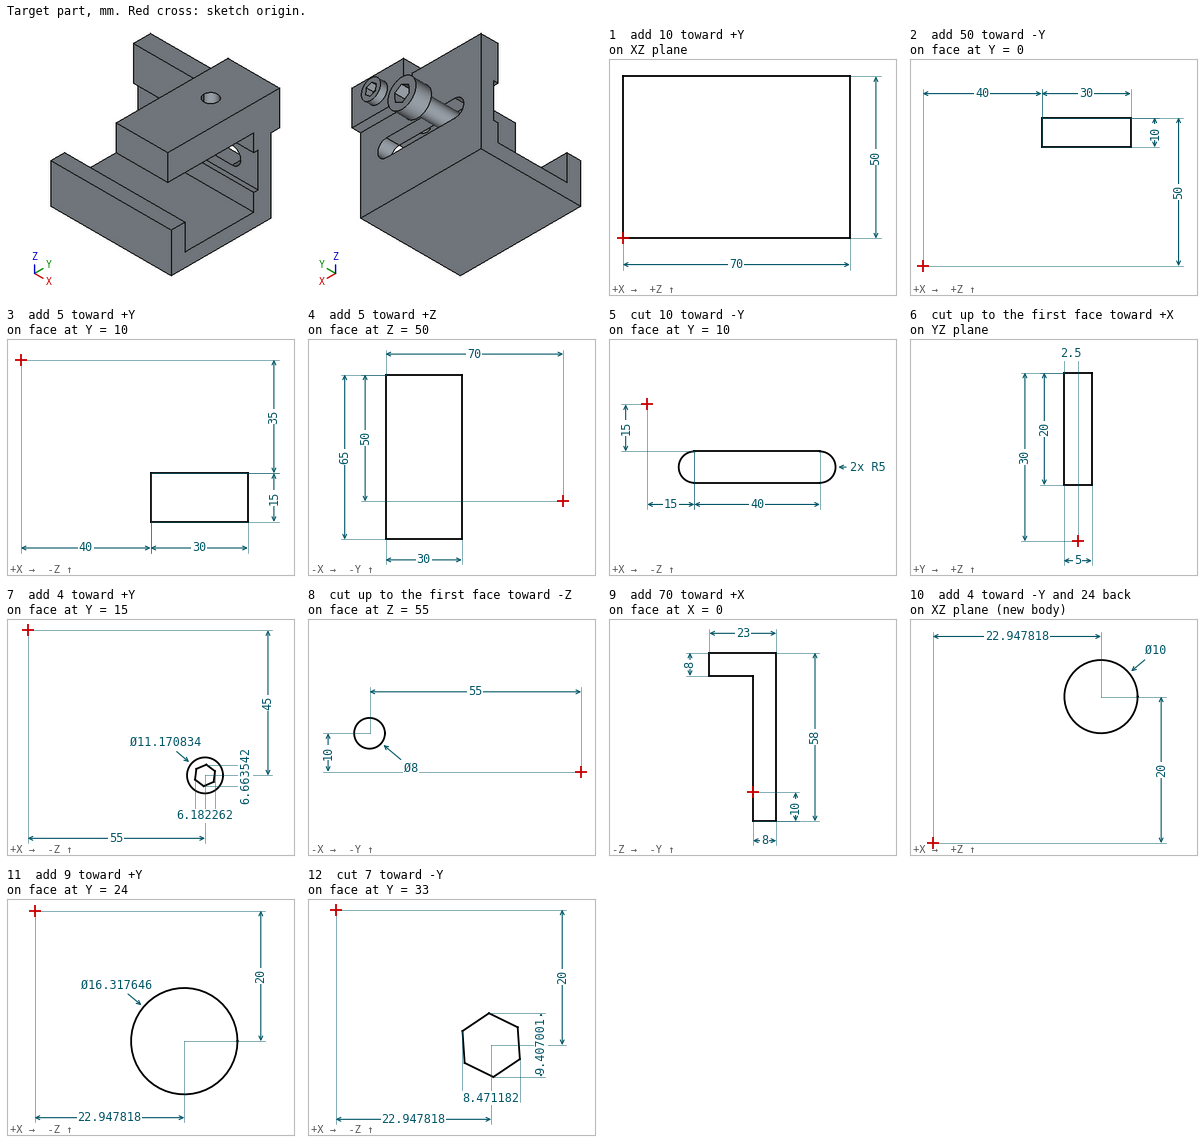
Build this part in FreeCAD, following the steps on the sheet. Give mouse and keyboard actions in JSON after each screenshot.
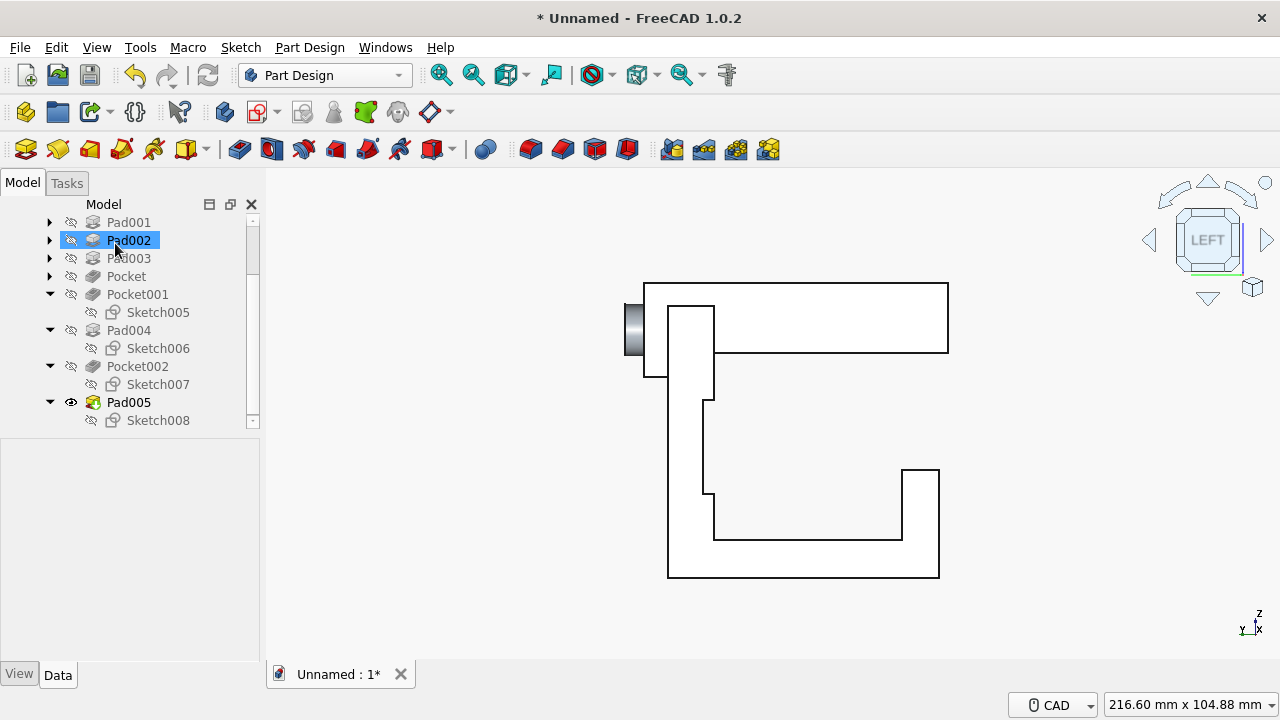
{"action": "left_click", "coordinate": [226, 112]}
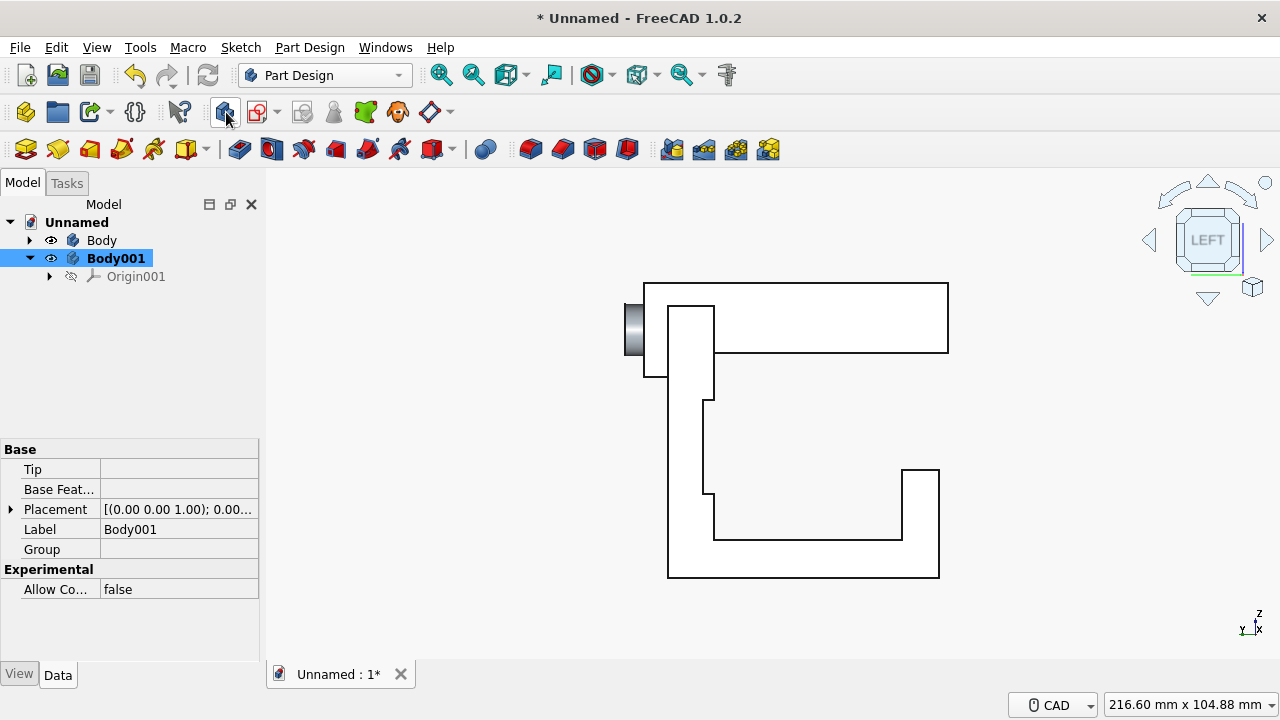
{"action": "left_click", "coordinate": [306, 619]}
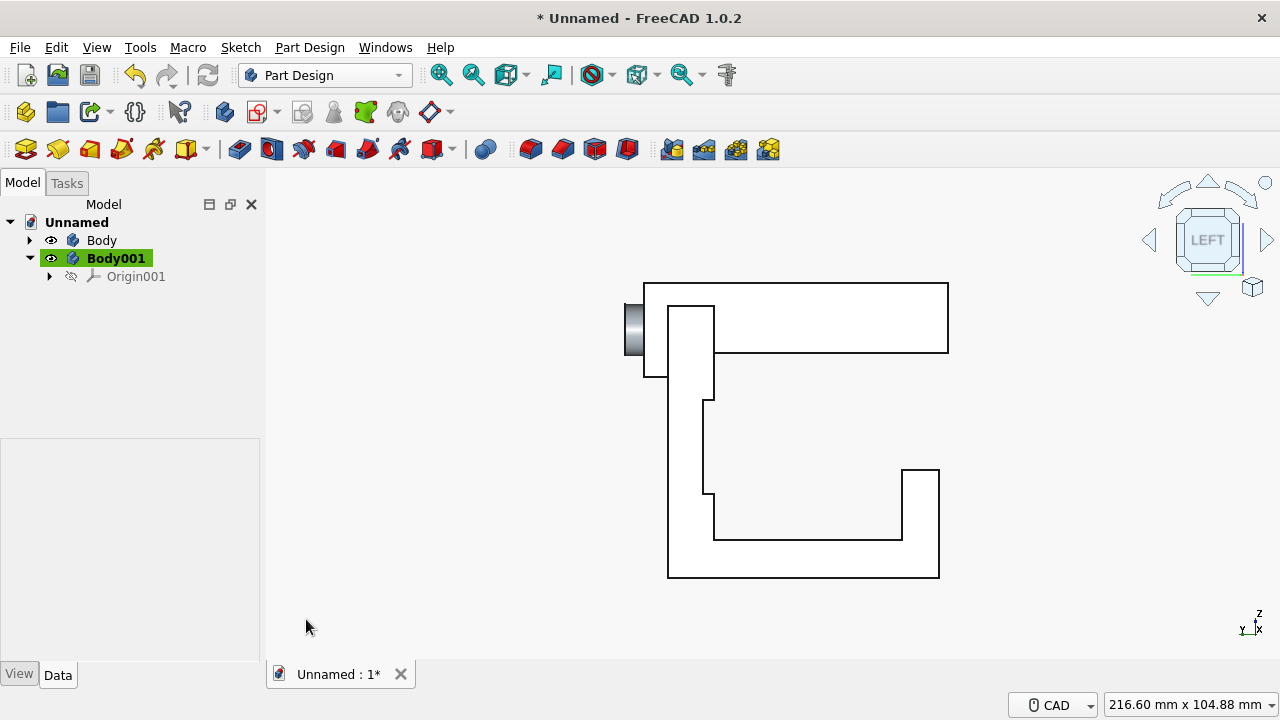
{"action": "left_click", "coordinate": [258, 112]}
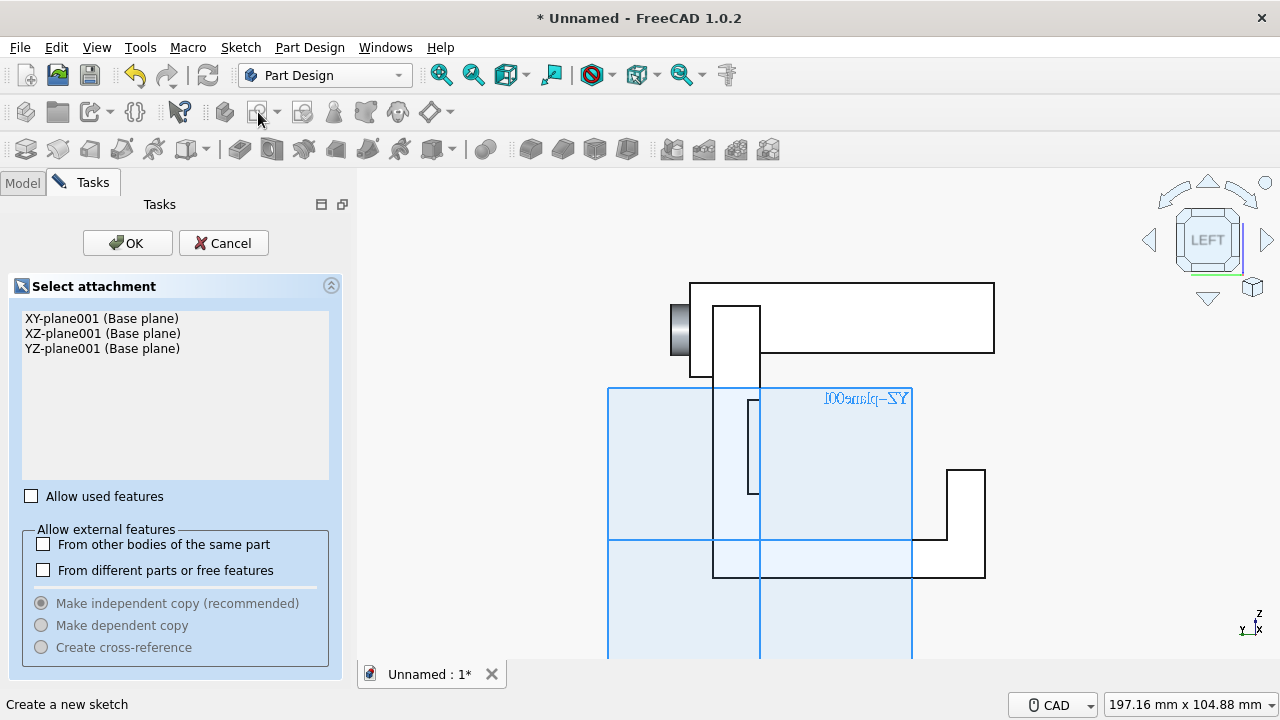
{"action": "left_click", "coordinate": [82, 334]}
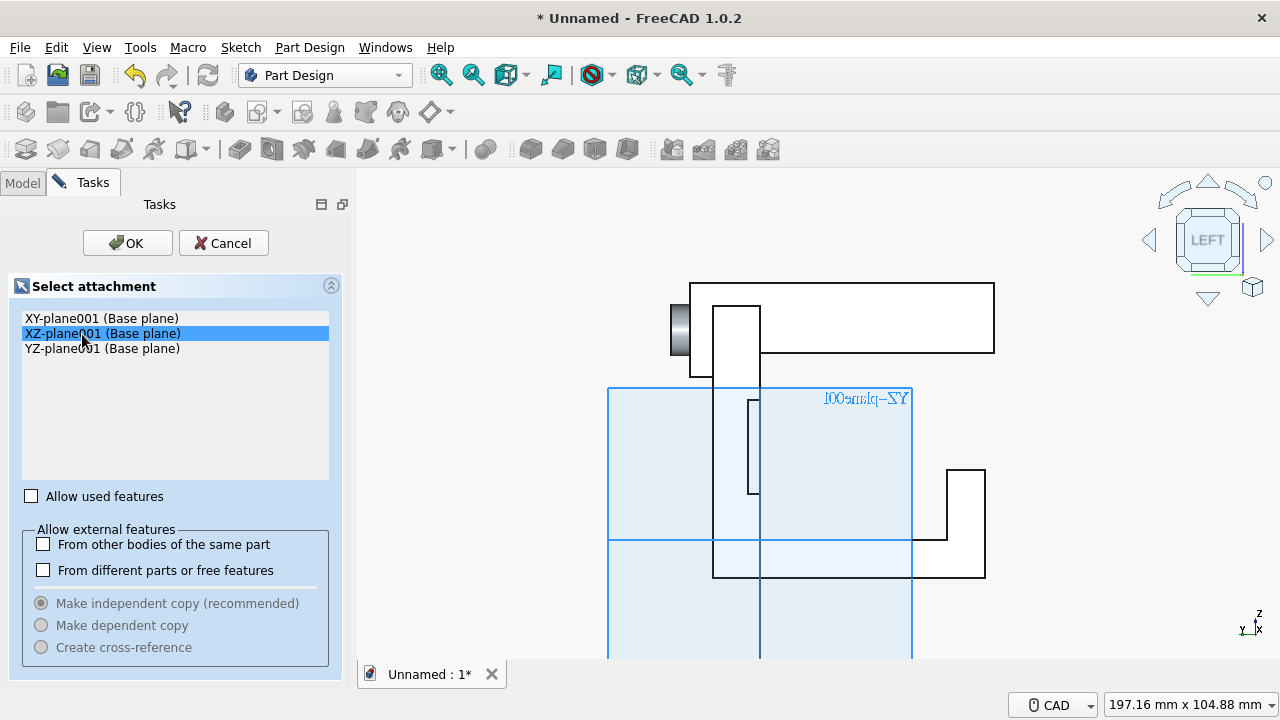
{"action": "left_click", "coordinate": [128, 243]}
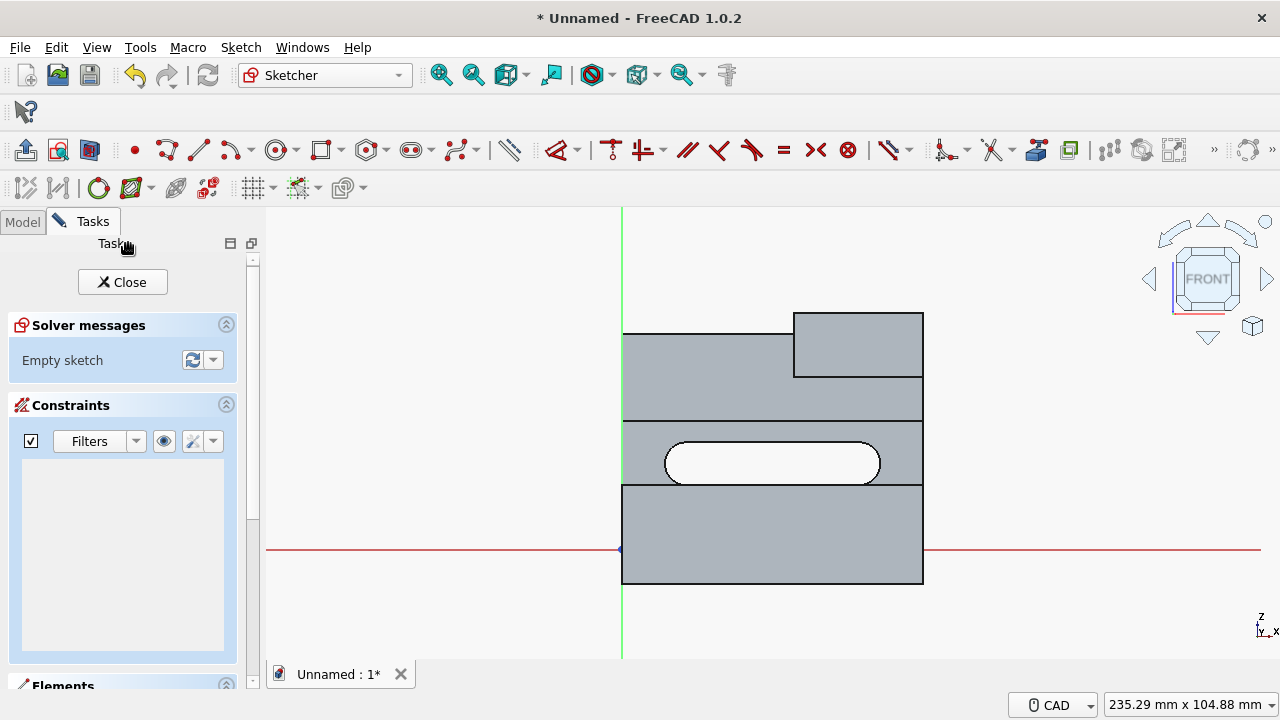
{"action": "scroll", "coordinate": [724, 470], "scroll_direction": "up", "scroll_amount": 9}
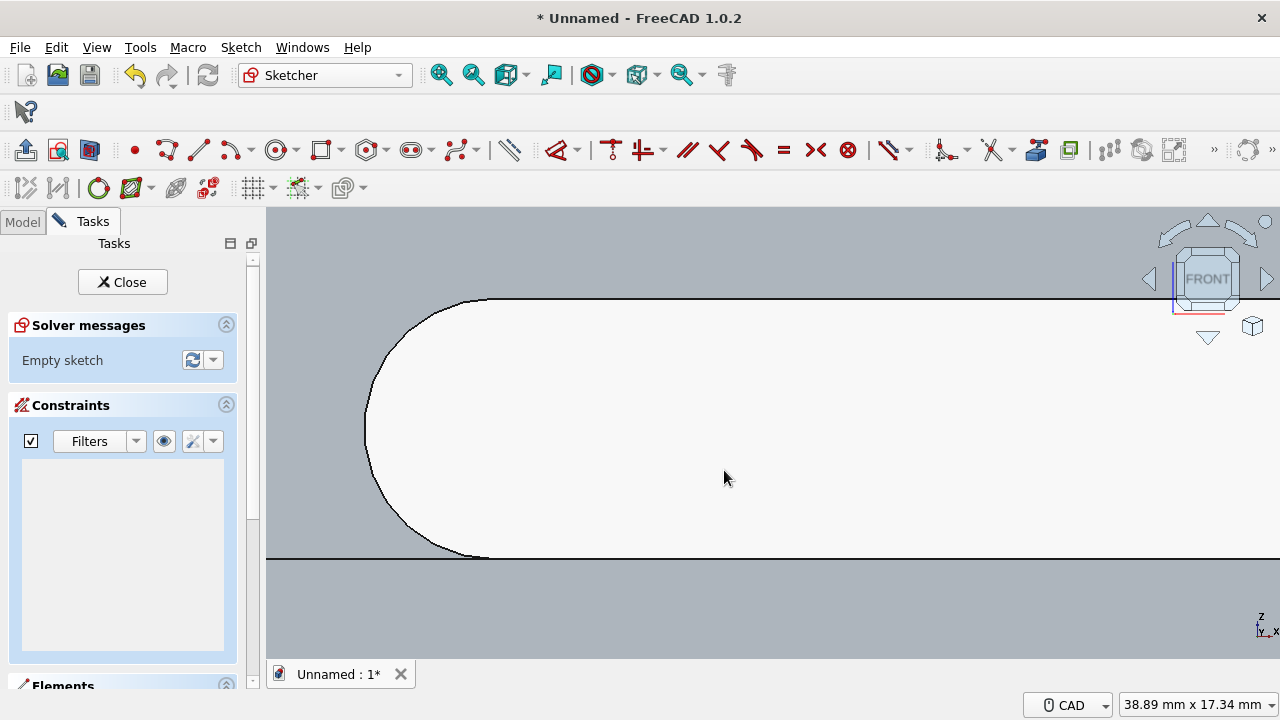
{"action": "left_click", "coordinate": [276, 150]}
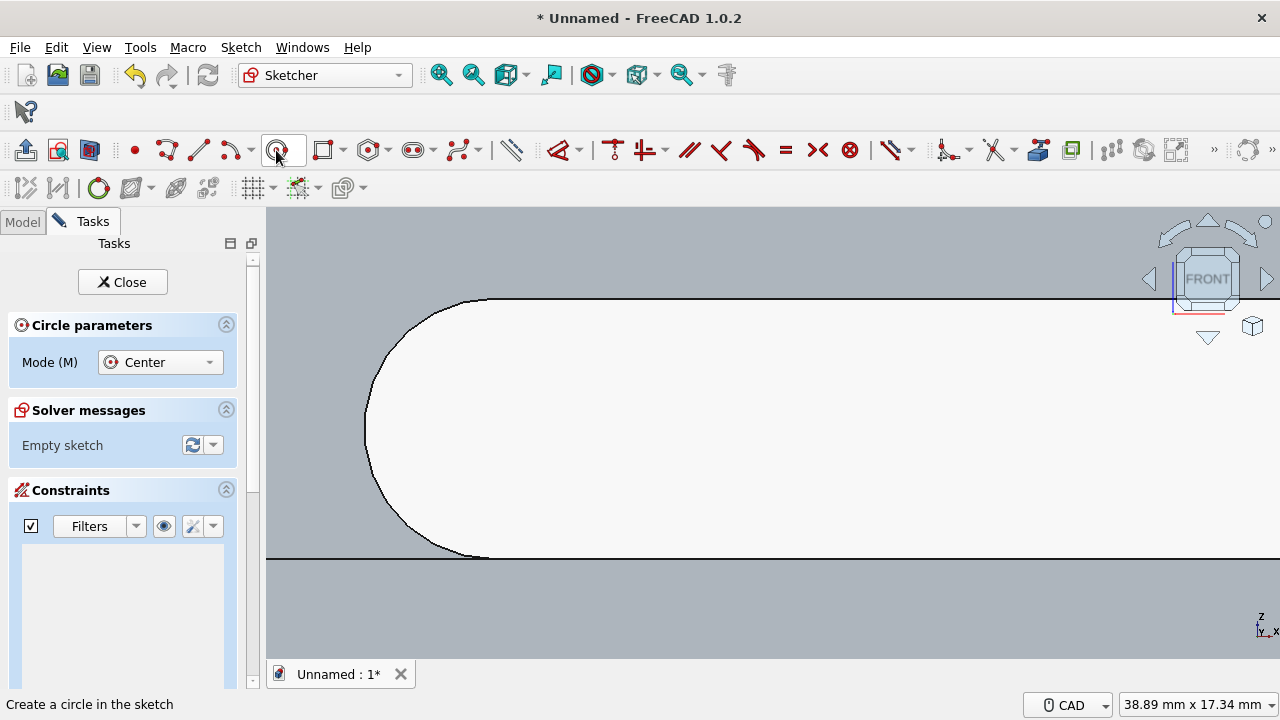
{"action": "left_click", "coordinate": [702, 429]}
{"action": "left_click", "coordinate": [794, 337]}
{"action": "key", "text": "Escape"}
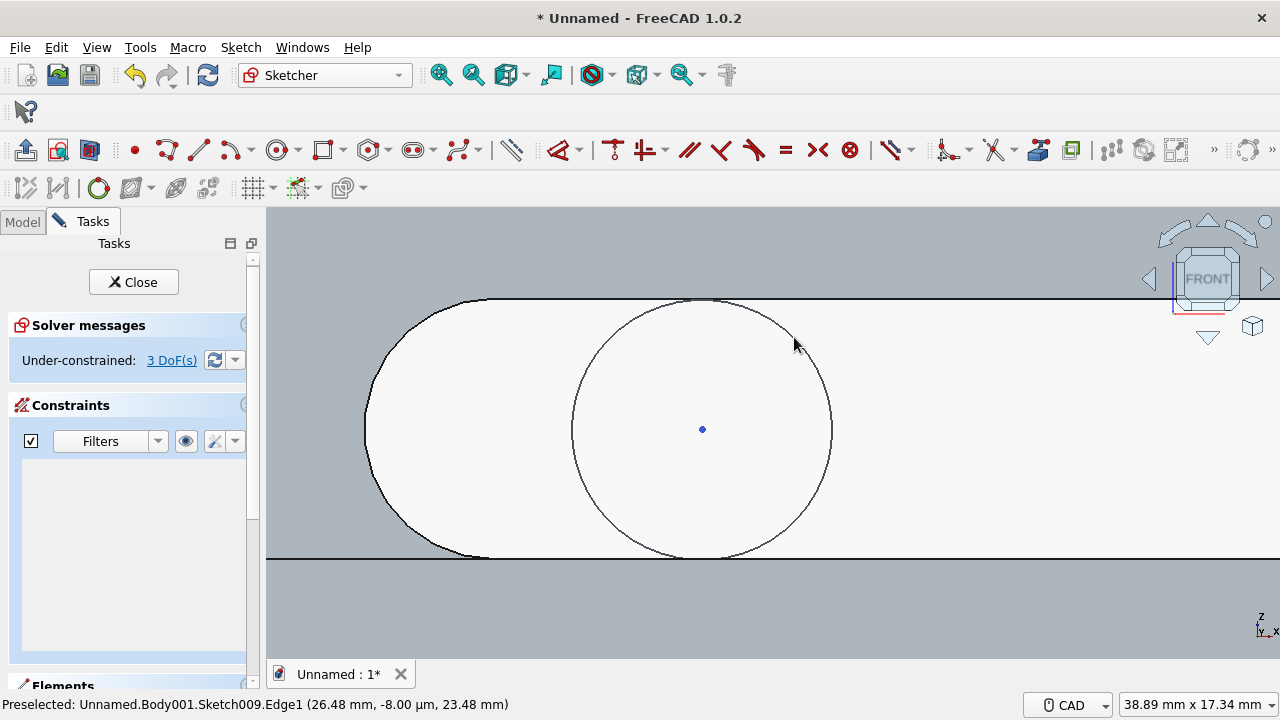
{"action": "left_click", "coordinate": [558, 150]}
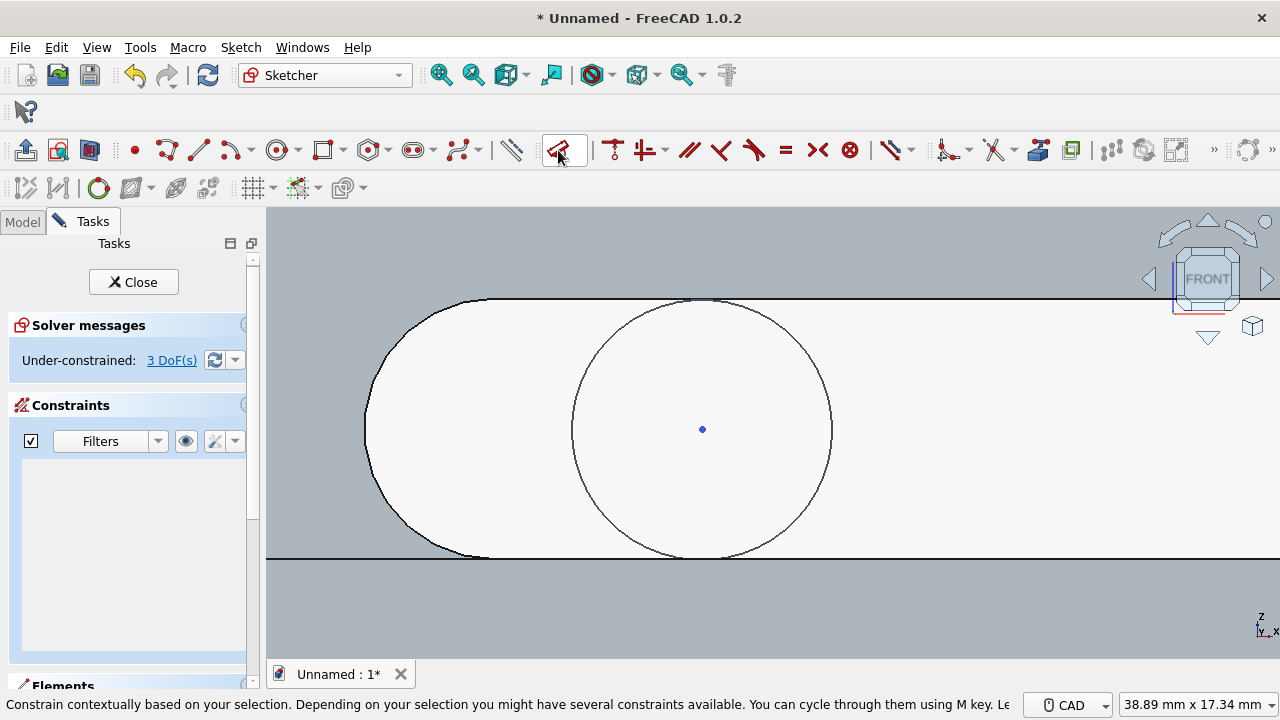
{"action": "left_click", "coordinate": [794, 338]}
{"action": "left_click", "coordinate": [817, 315]}